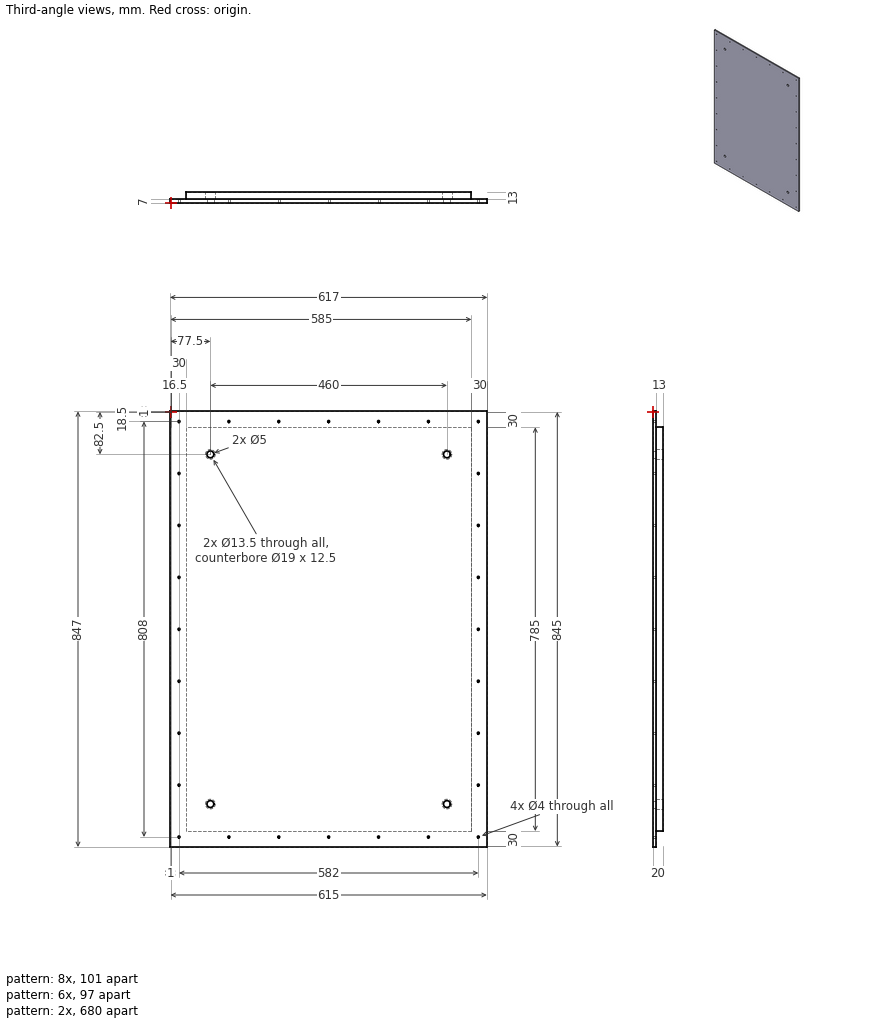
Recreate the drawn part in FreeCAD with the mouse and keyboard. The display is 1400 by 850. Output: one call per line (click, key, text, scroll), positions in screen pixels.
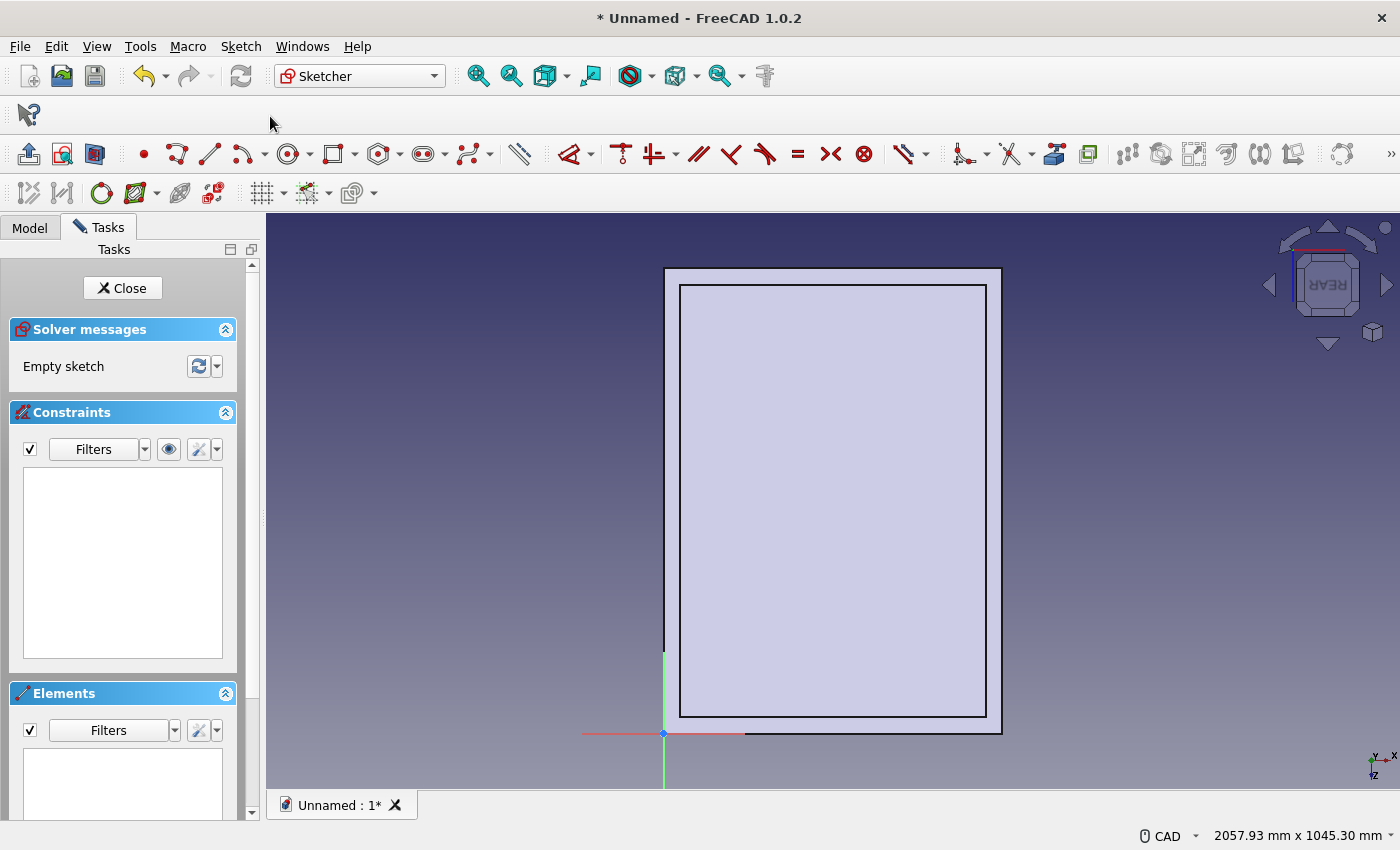
click(95, 154)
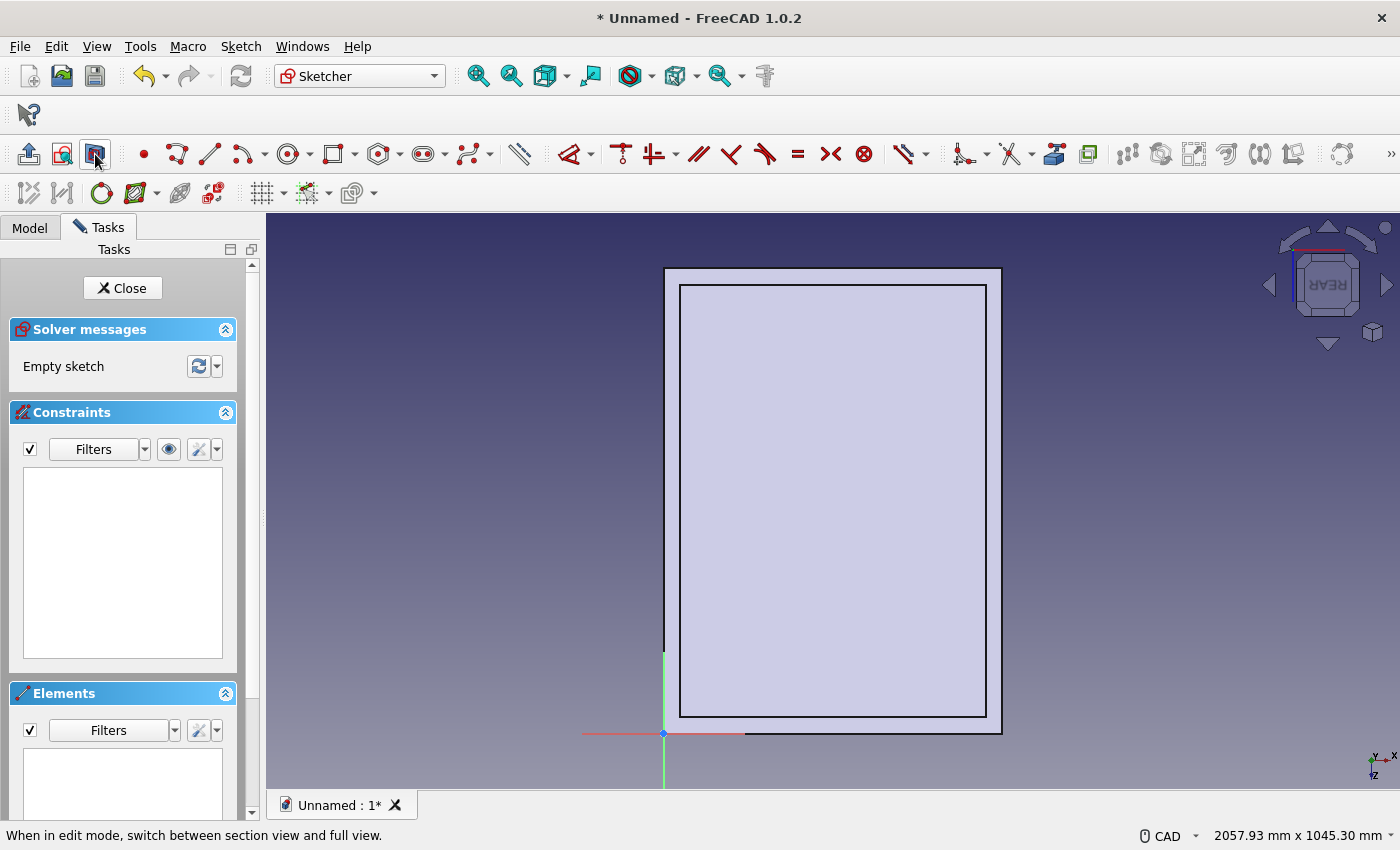
click(288, 154)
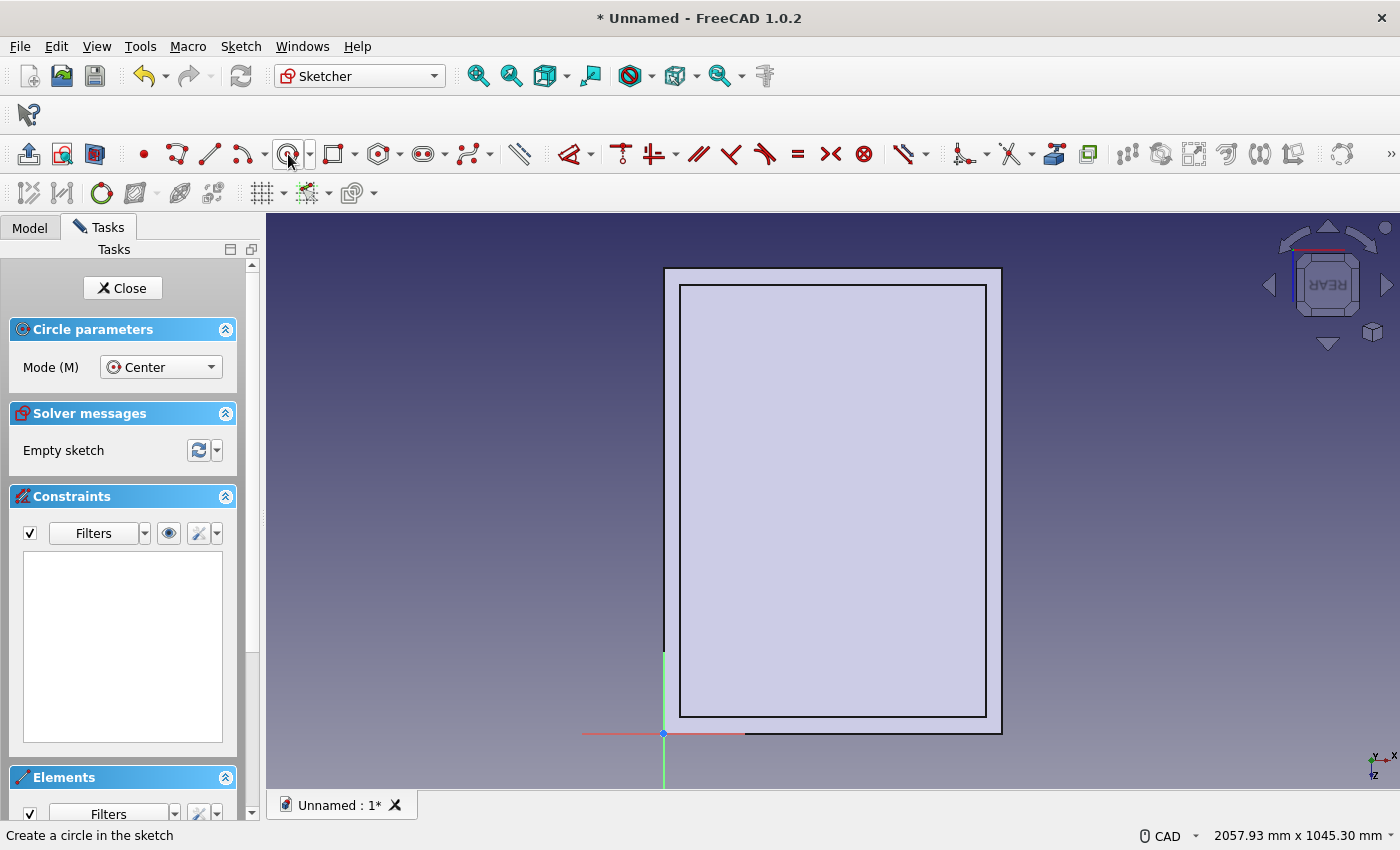
scroll(993, 278, up, 16)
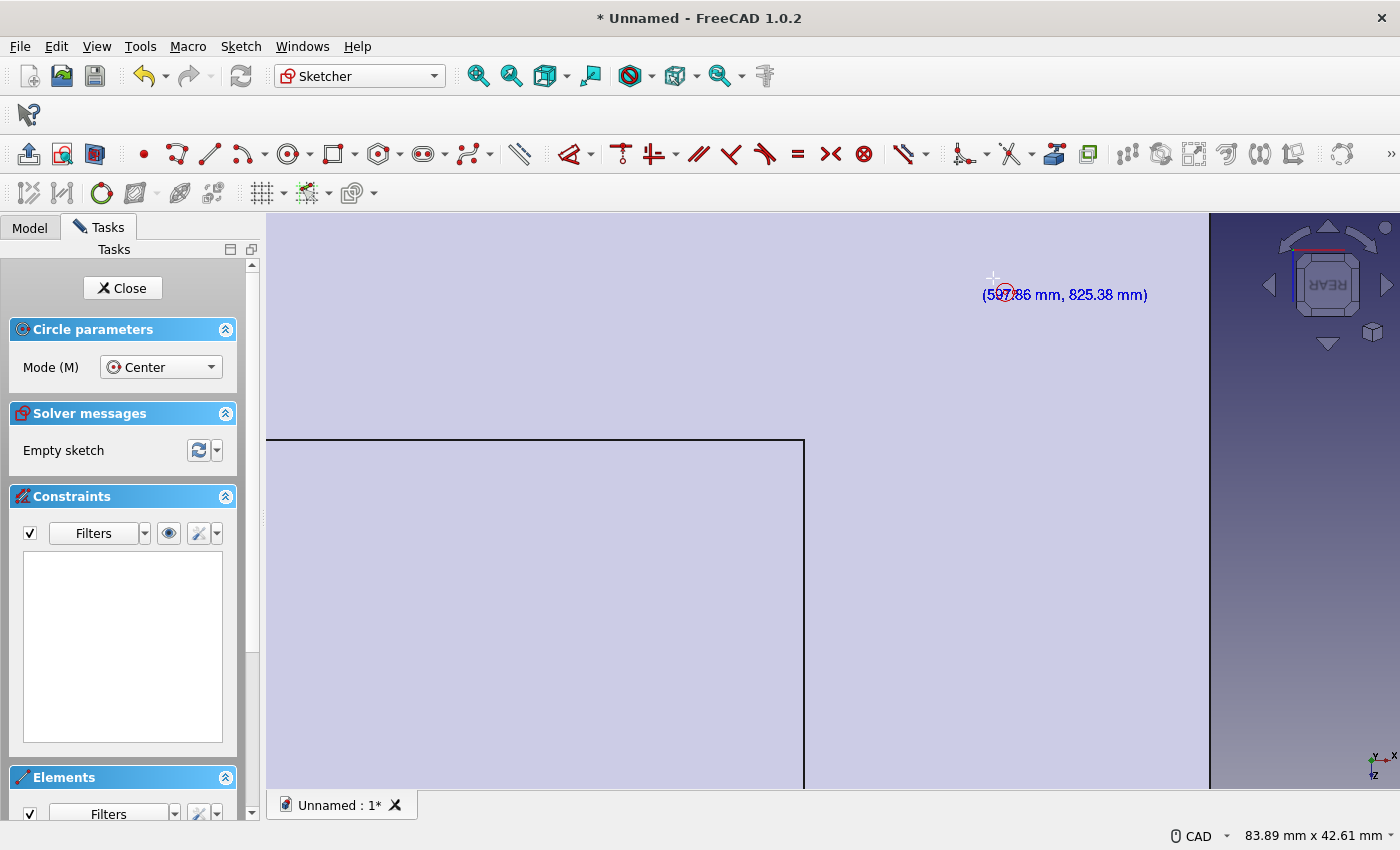
scroll(926, 273, down, 16)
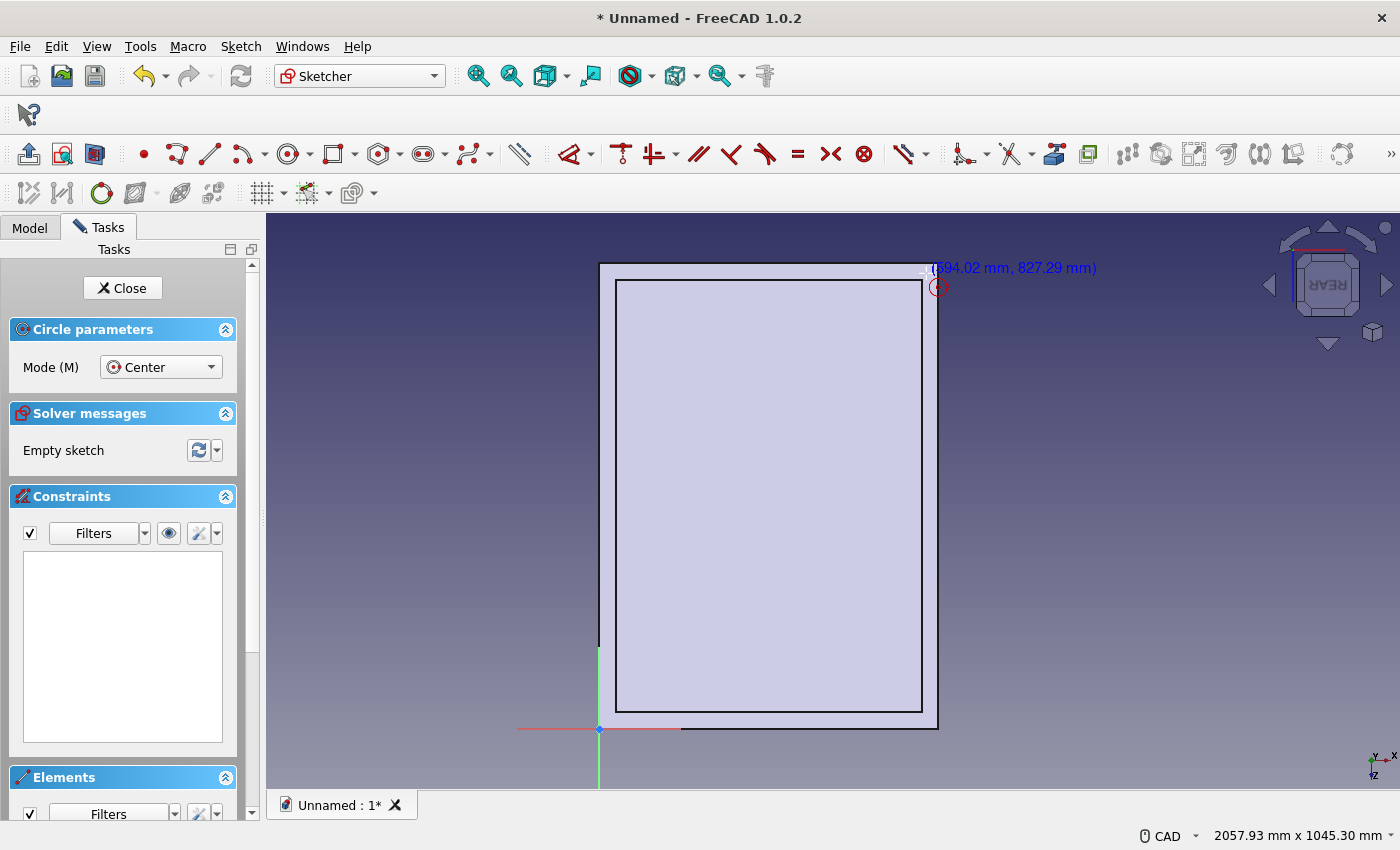
click(929, 274)
move(930, 273)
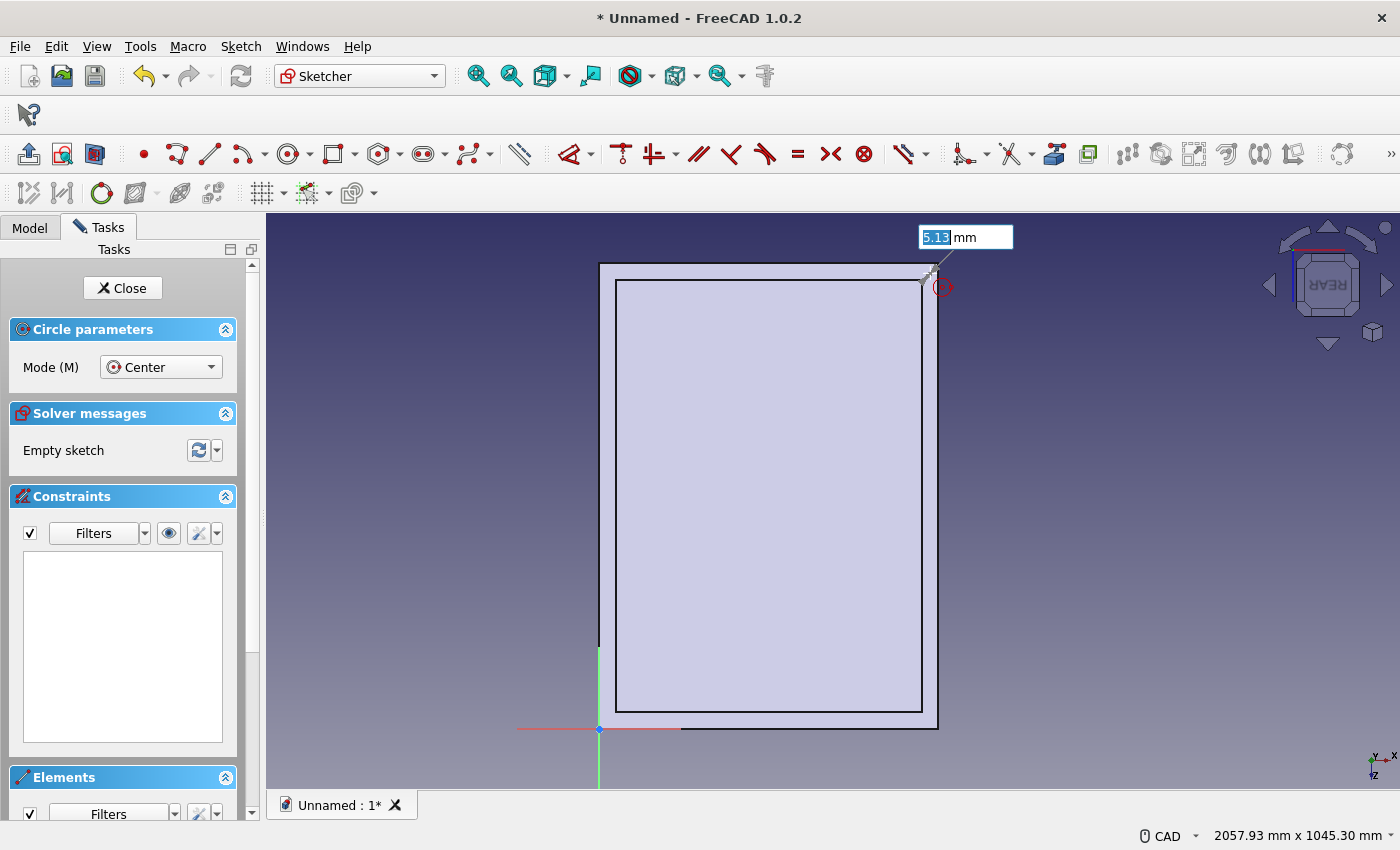
text(4)
key(Return)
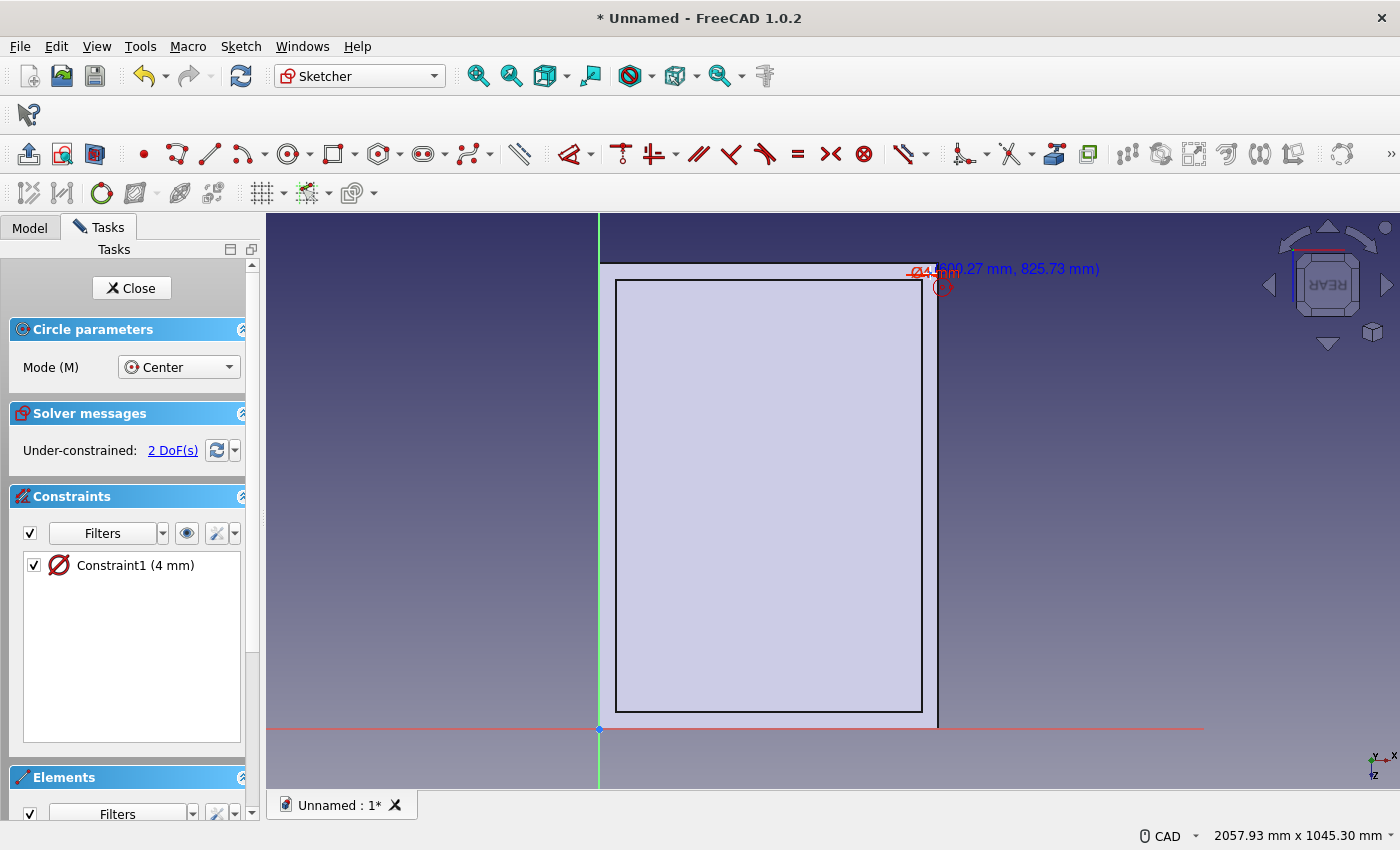
scroll(608, 274, up, 16)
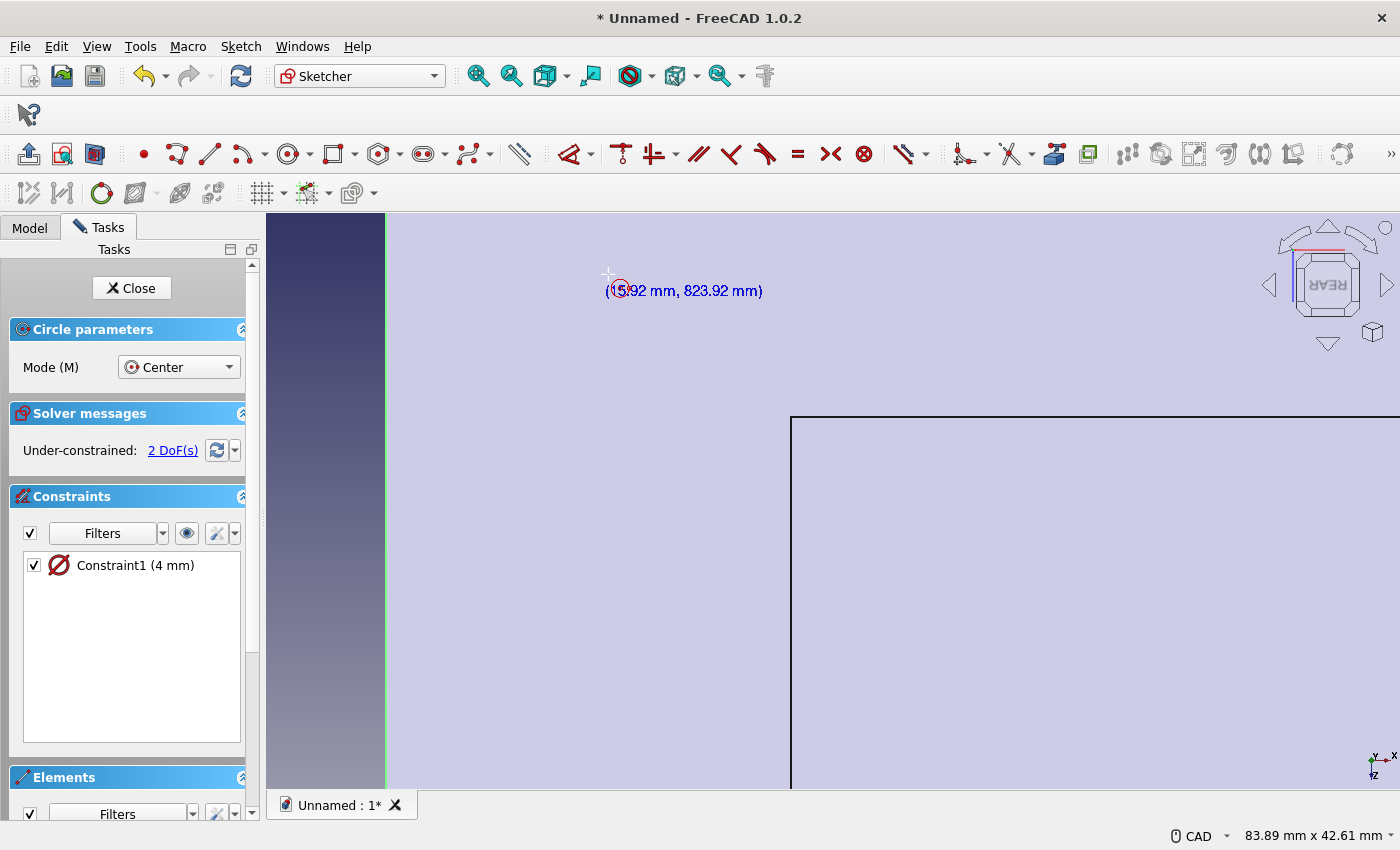
scroll(608, 274, down, 16)